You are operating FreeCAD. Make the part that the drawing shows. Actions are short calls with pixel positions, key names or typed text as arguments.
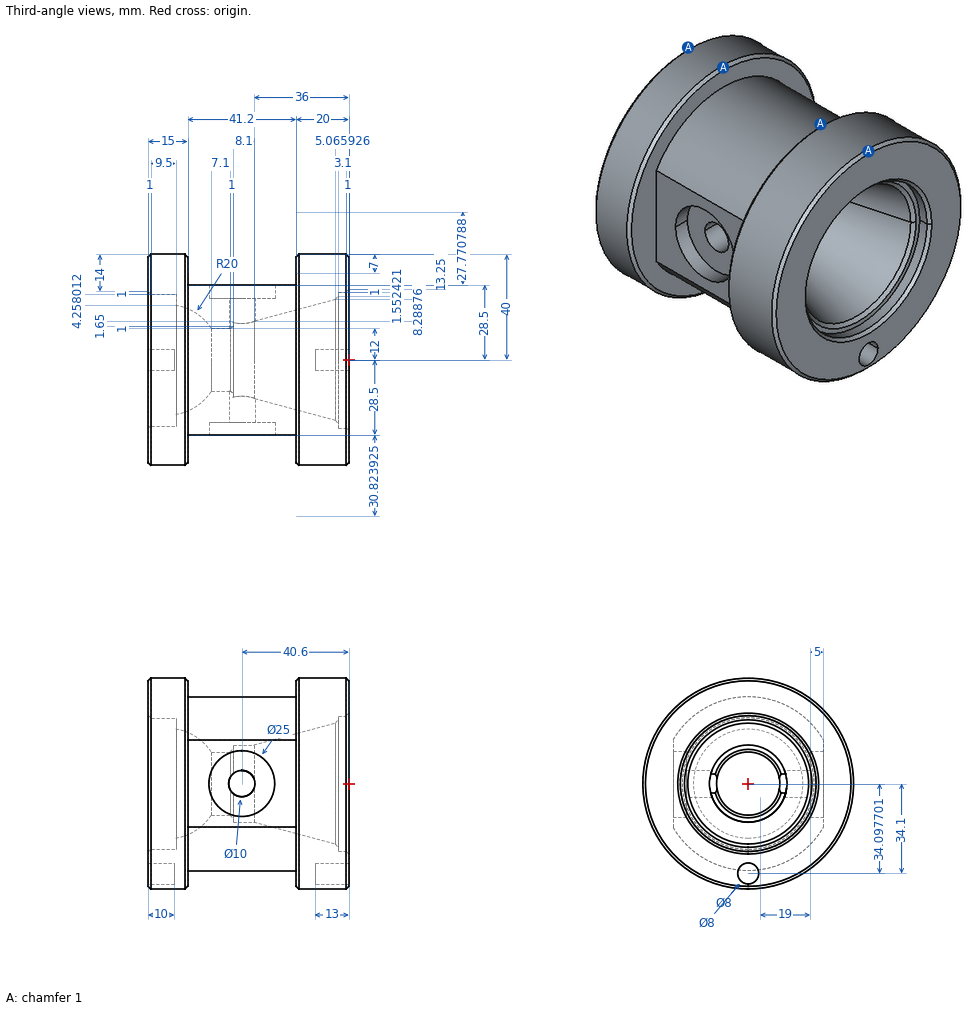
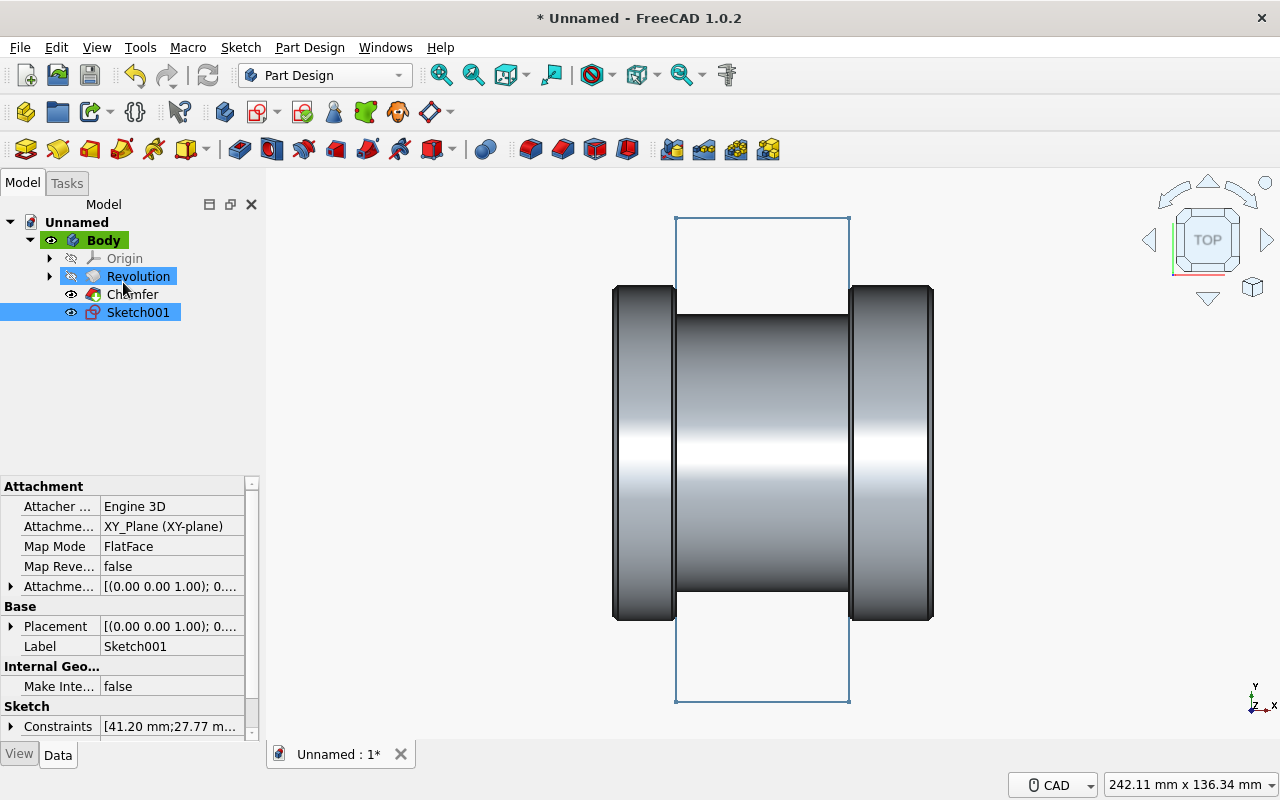
click(240, 150)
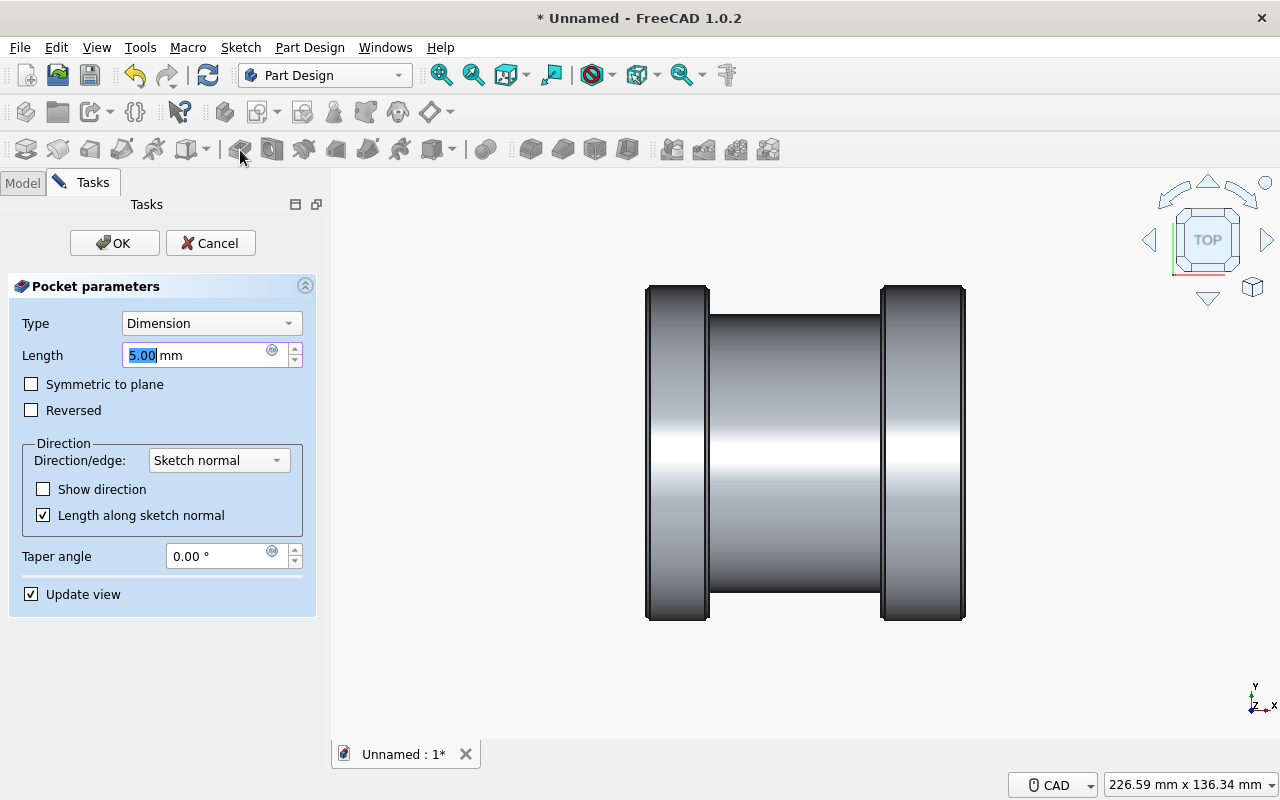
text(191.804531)
key(Tab)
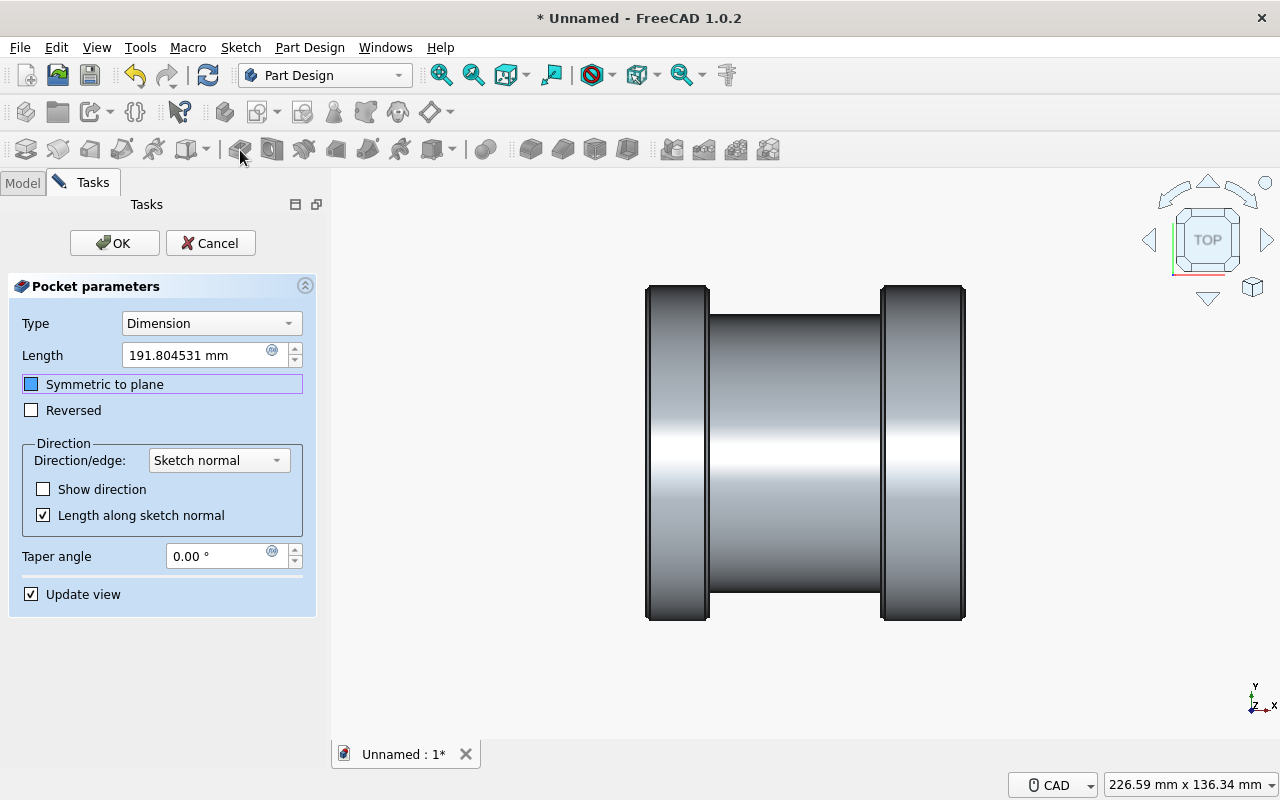
click(30, 384)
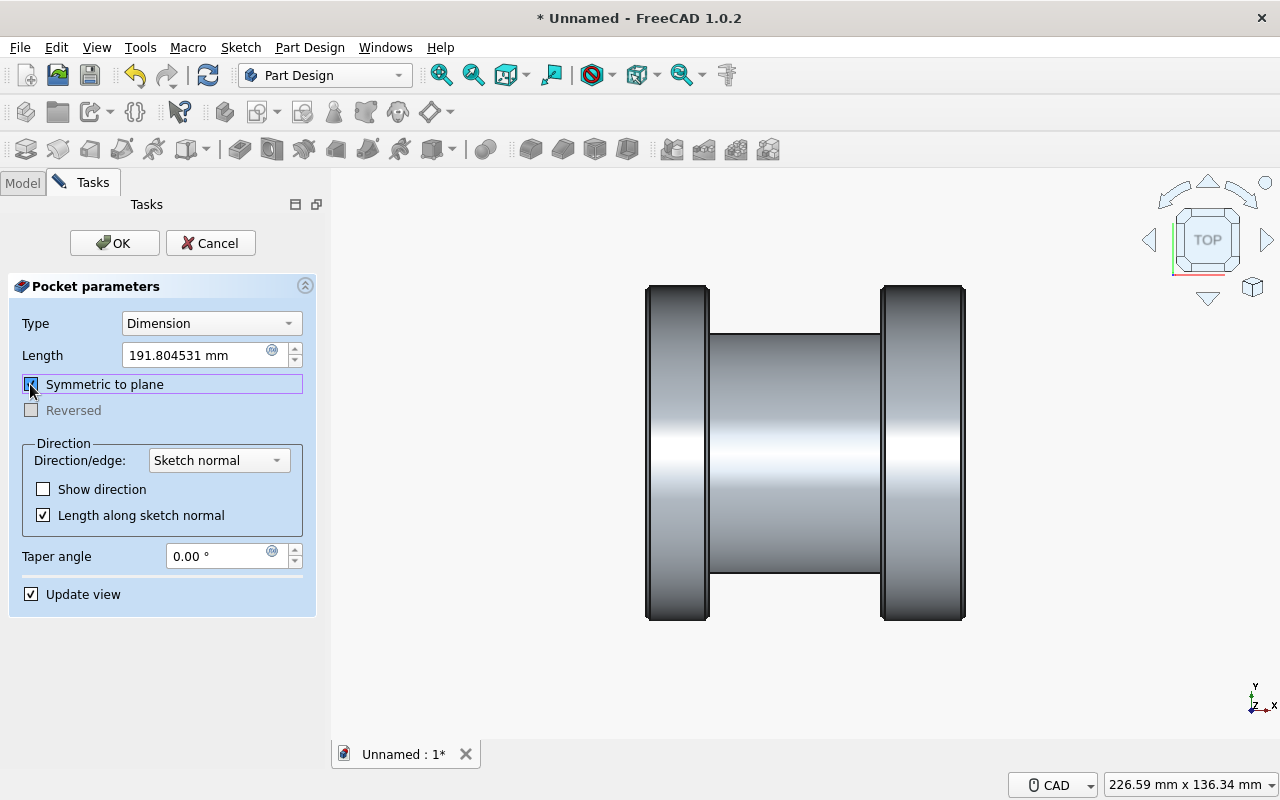
click(115, 243)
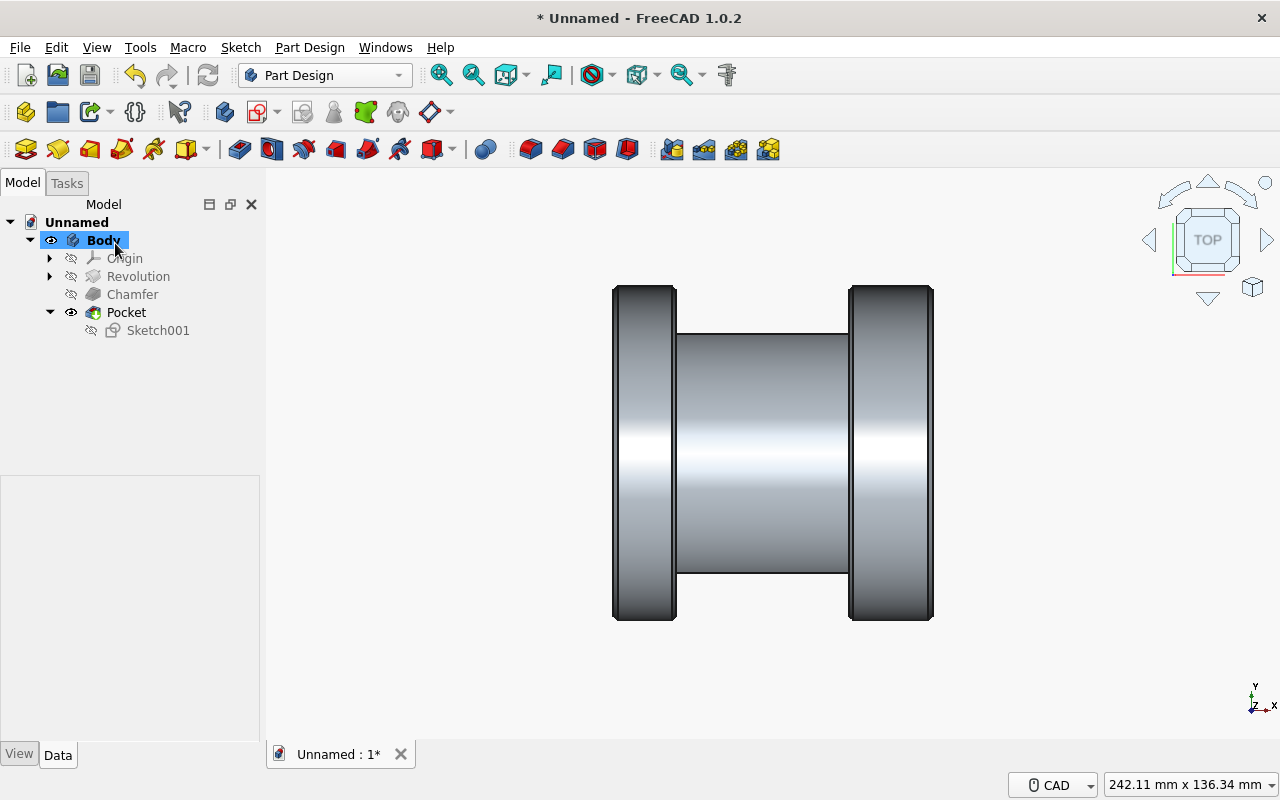
key(4)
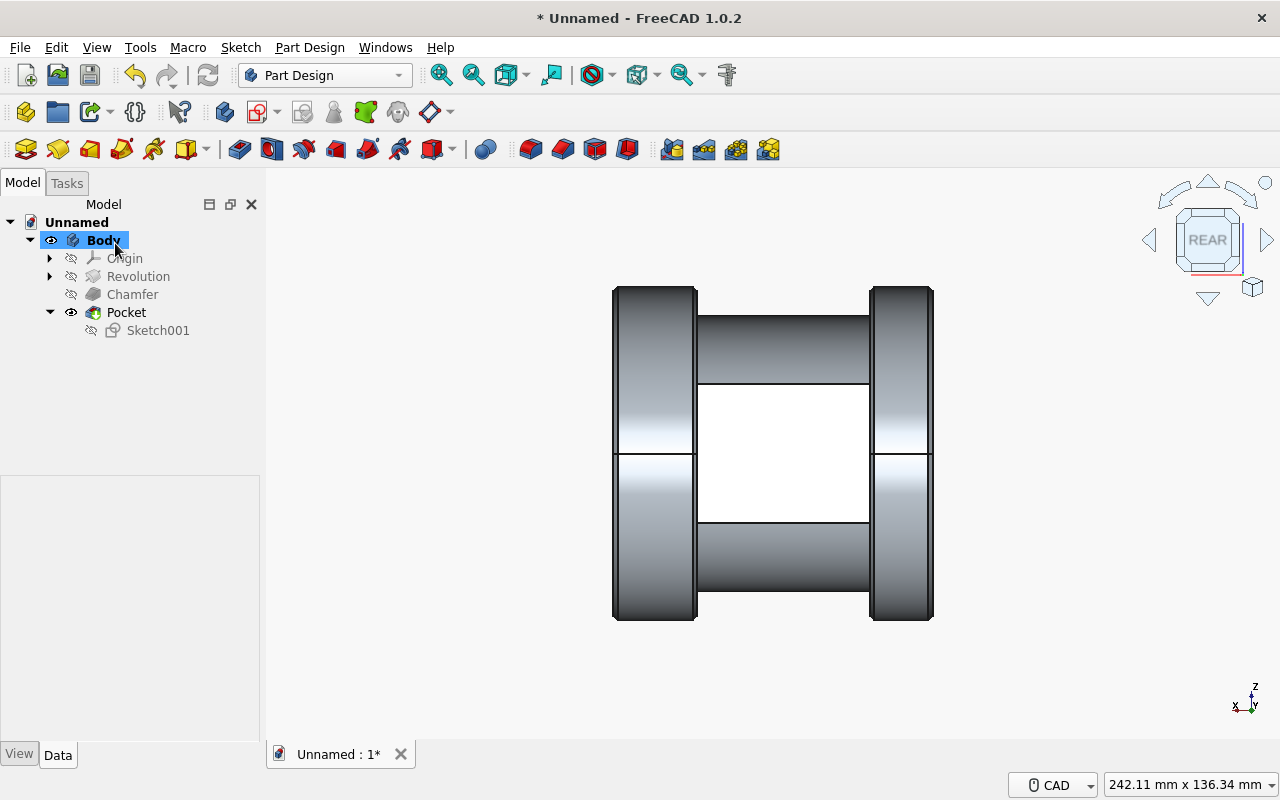
click(783, 452)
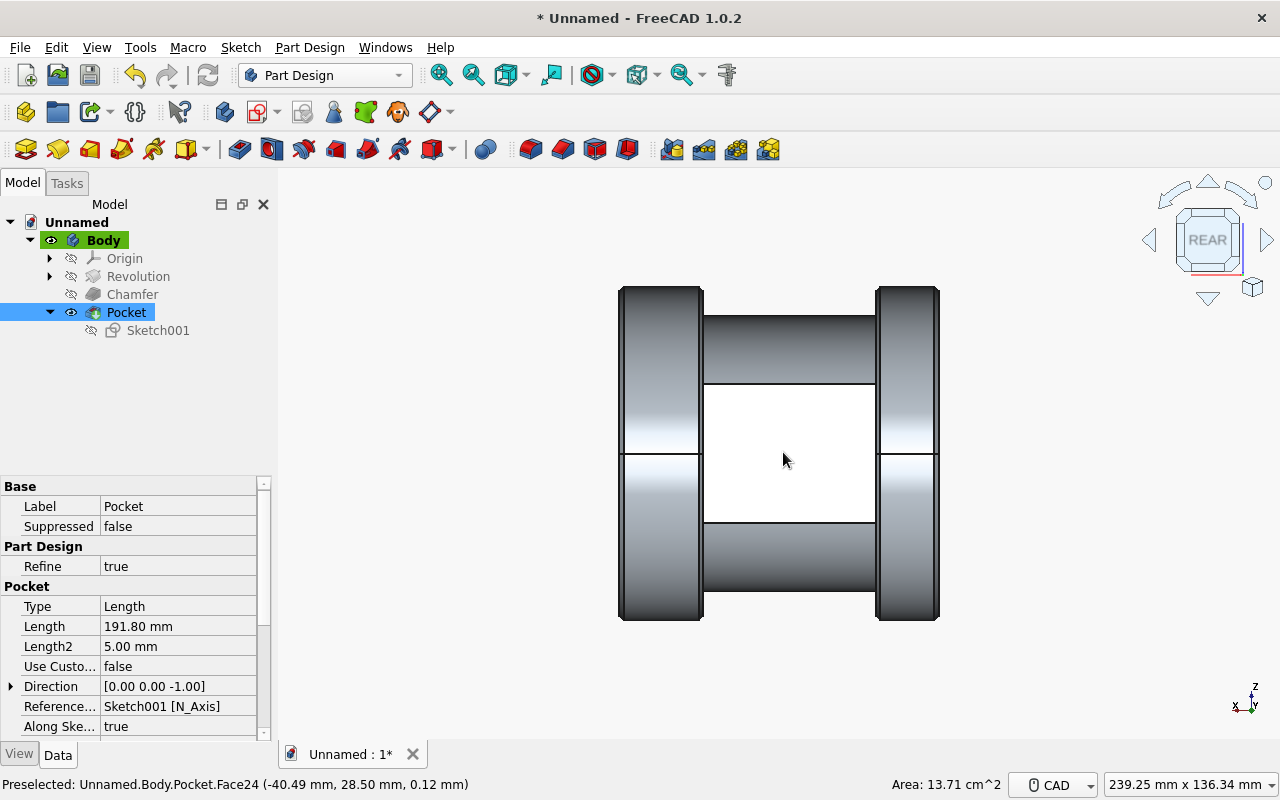
click(258, 112)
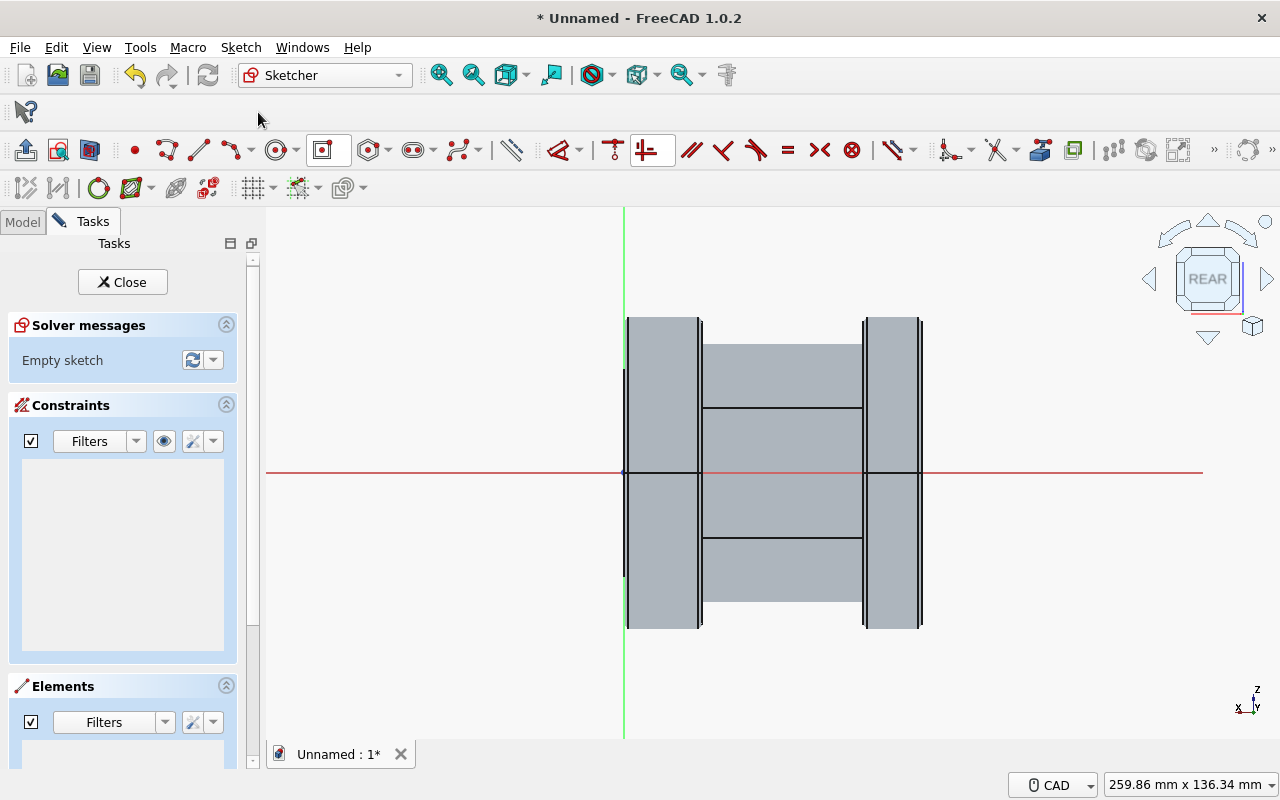
click(90, 150)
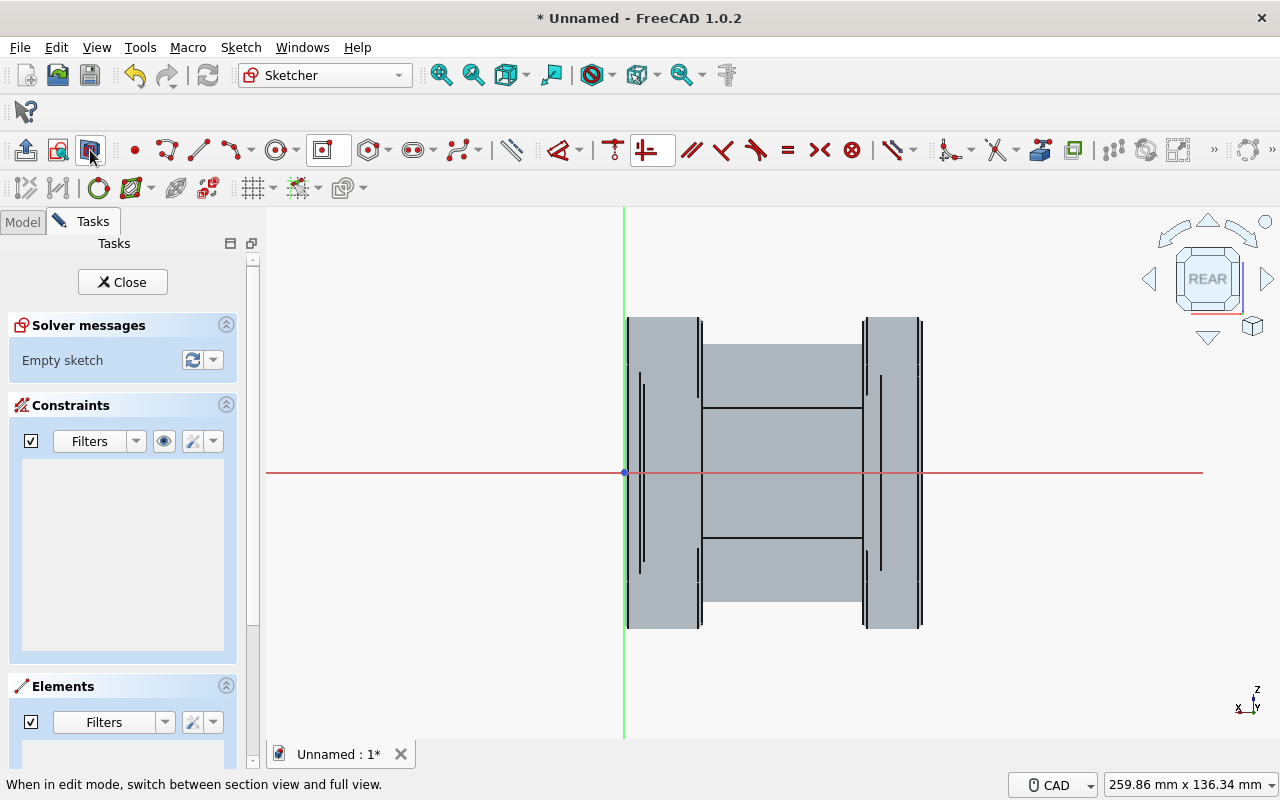
scroll(742, 473, up, 5)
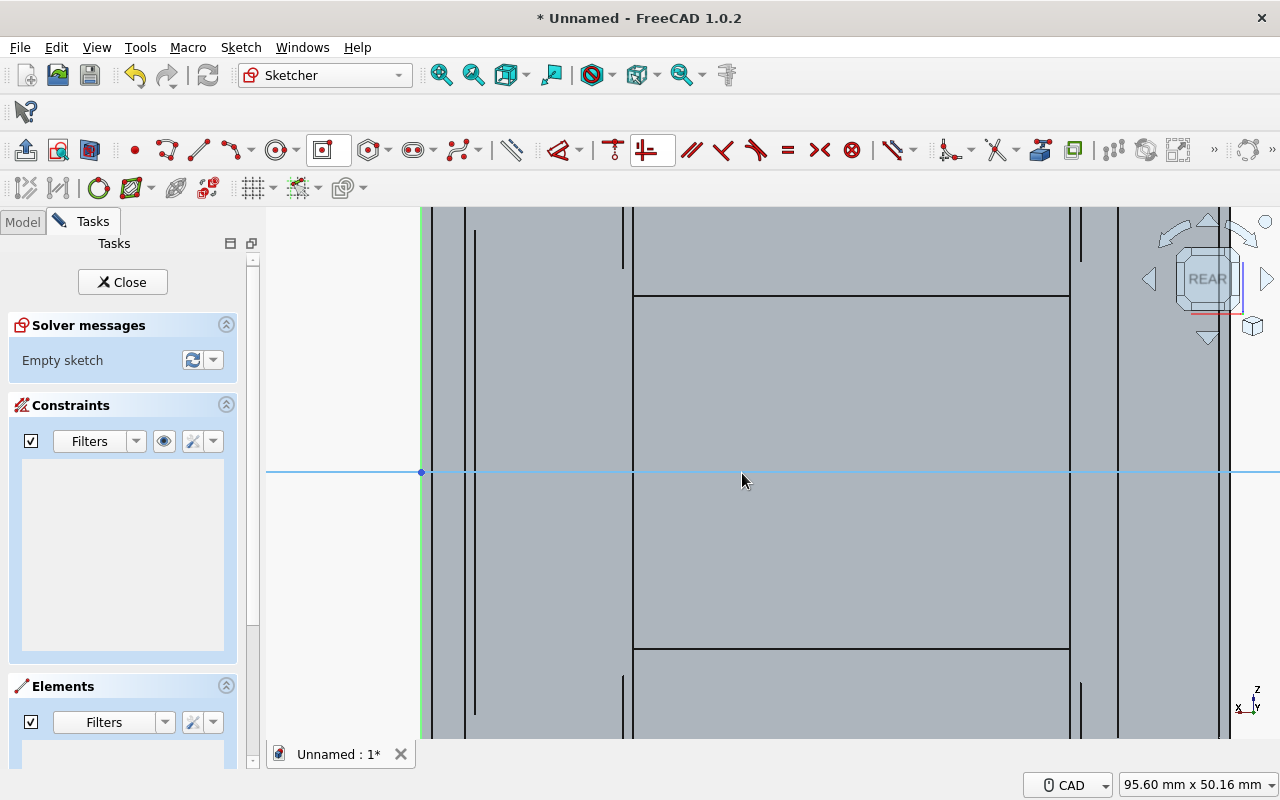
key(g)
key(c)